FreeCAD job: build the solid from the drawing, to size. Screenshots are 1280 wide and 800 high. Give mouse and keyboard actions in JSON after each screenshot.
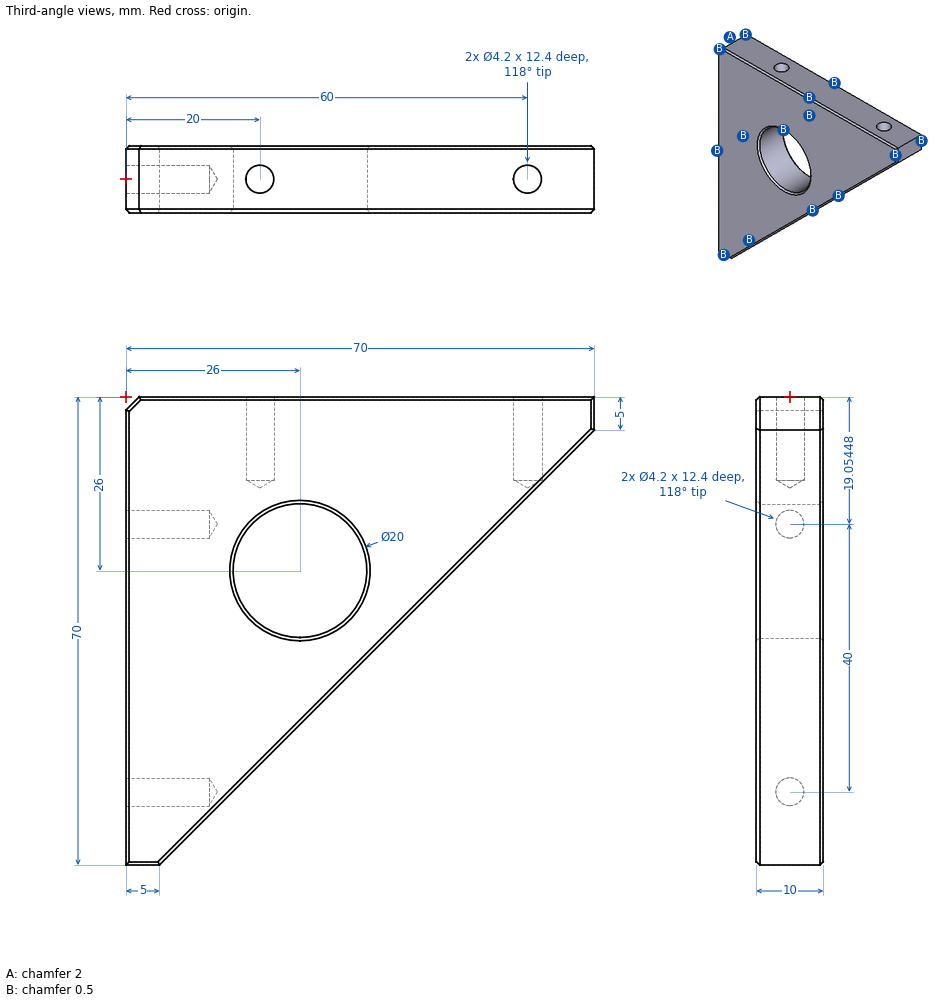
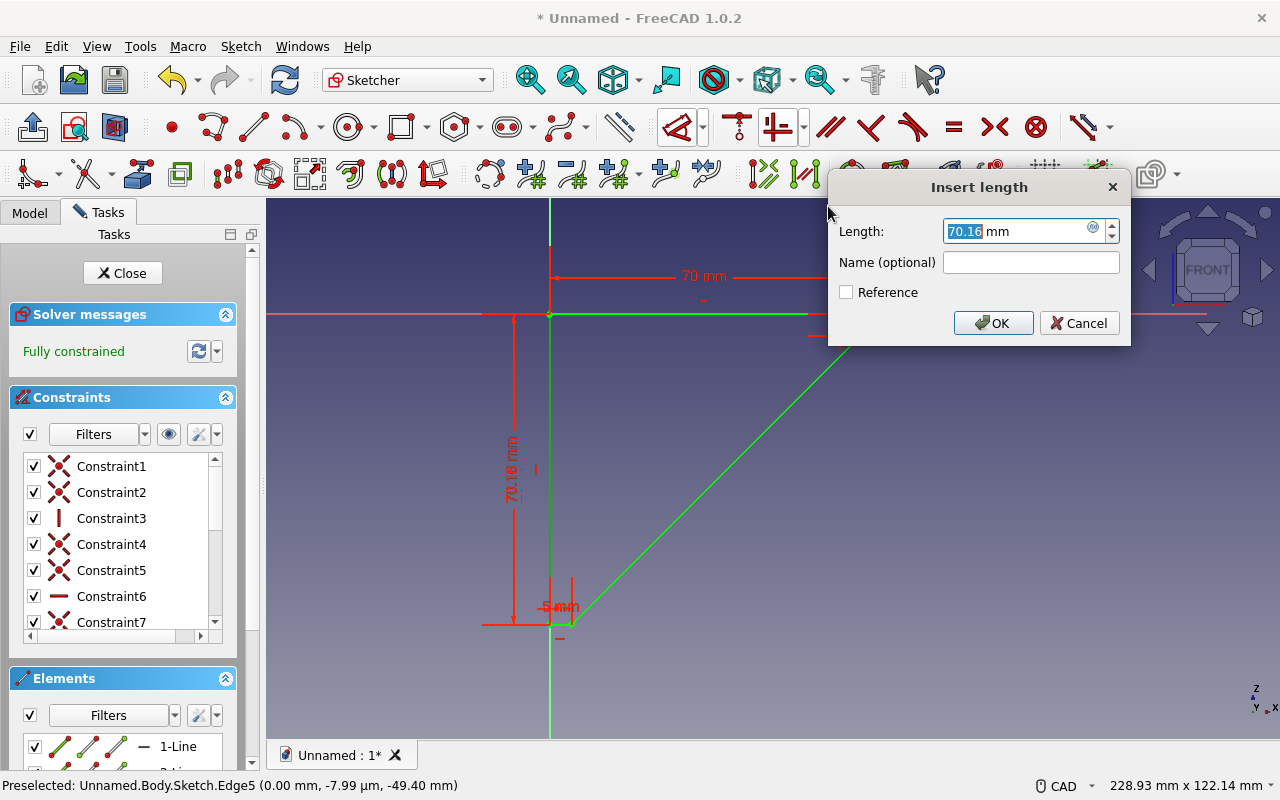
{"action": "type", "text": "70"}
{"action": "key", "text": "Return"}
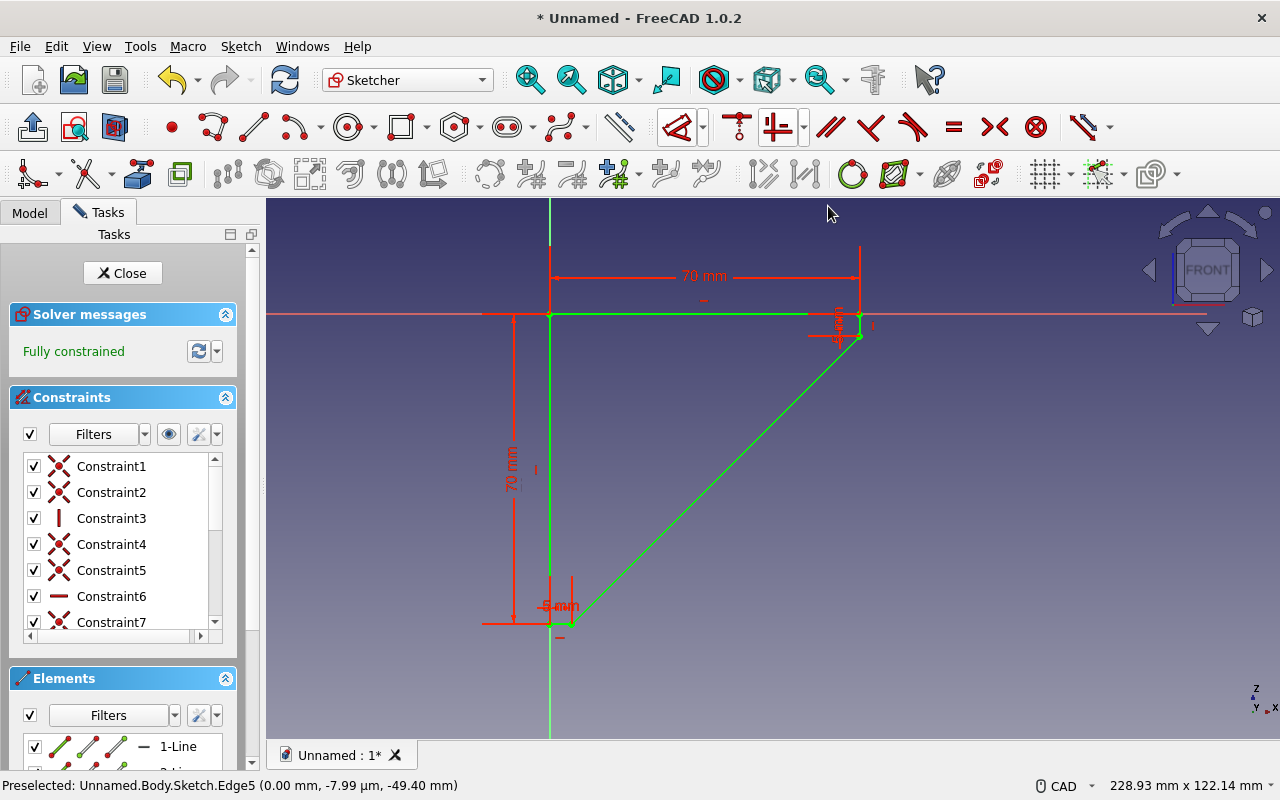
{"action": "left_click", "coordinate": [123, 273]}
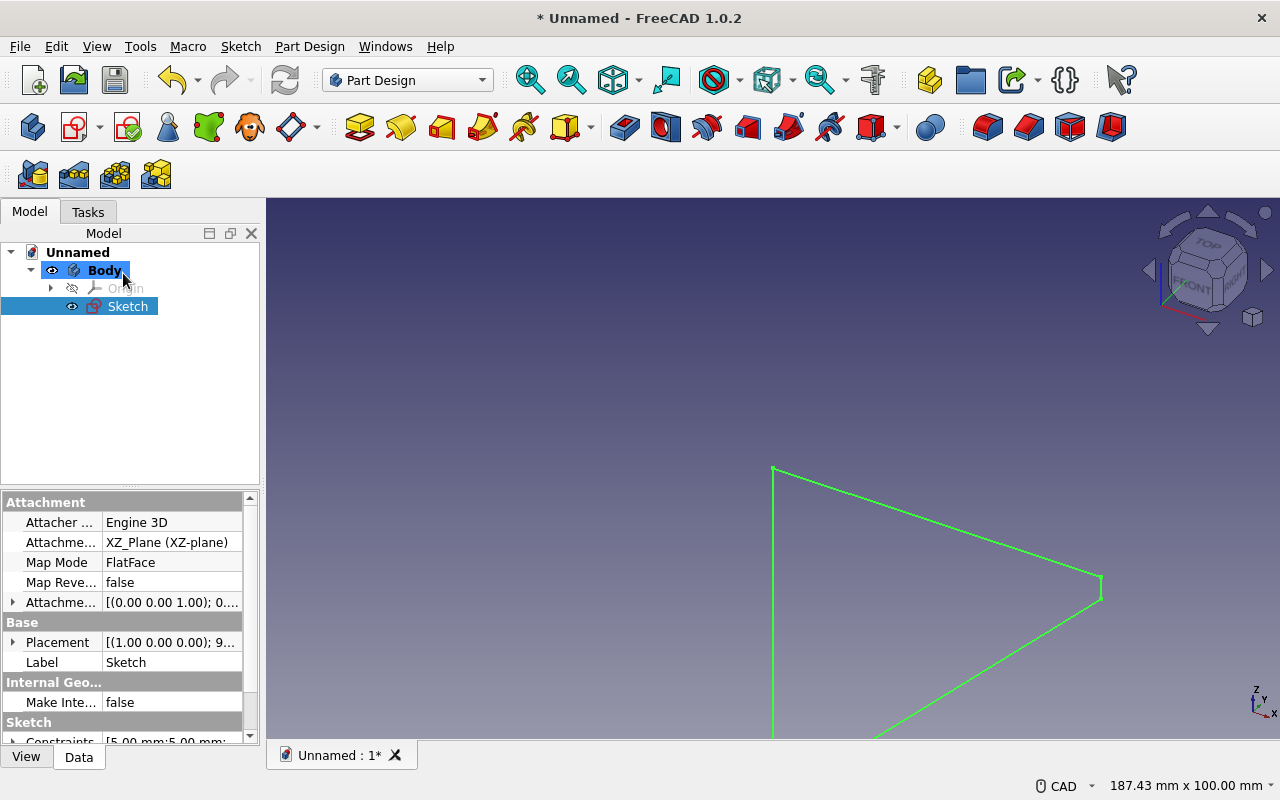
{"action": "left_click", "coordinate": [360, 128]}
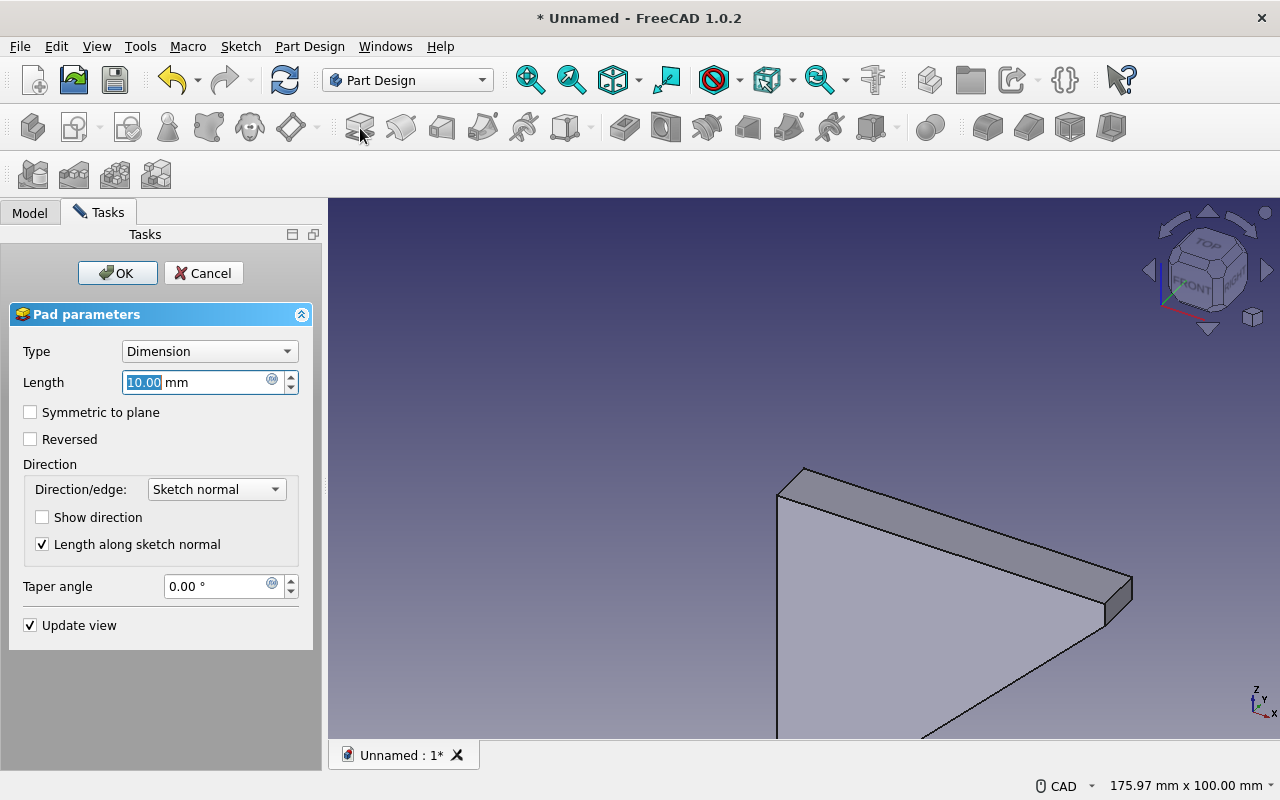
{"action": "type", "text": "10"}
{"action": "key", "text": "Tab"}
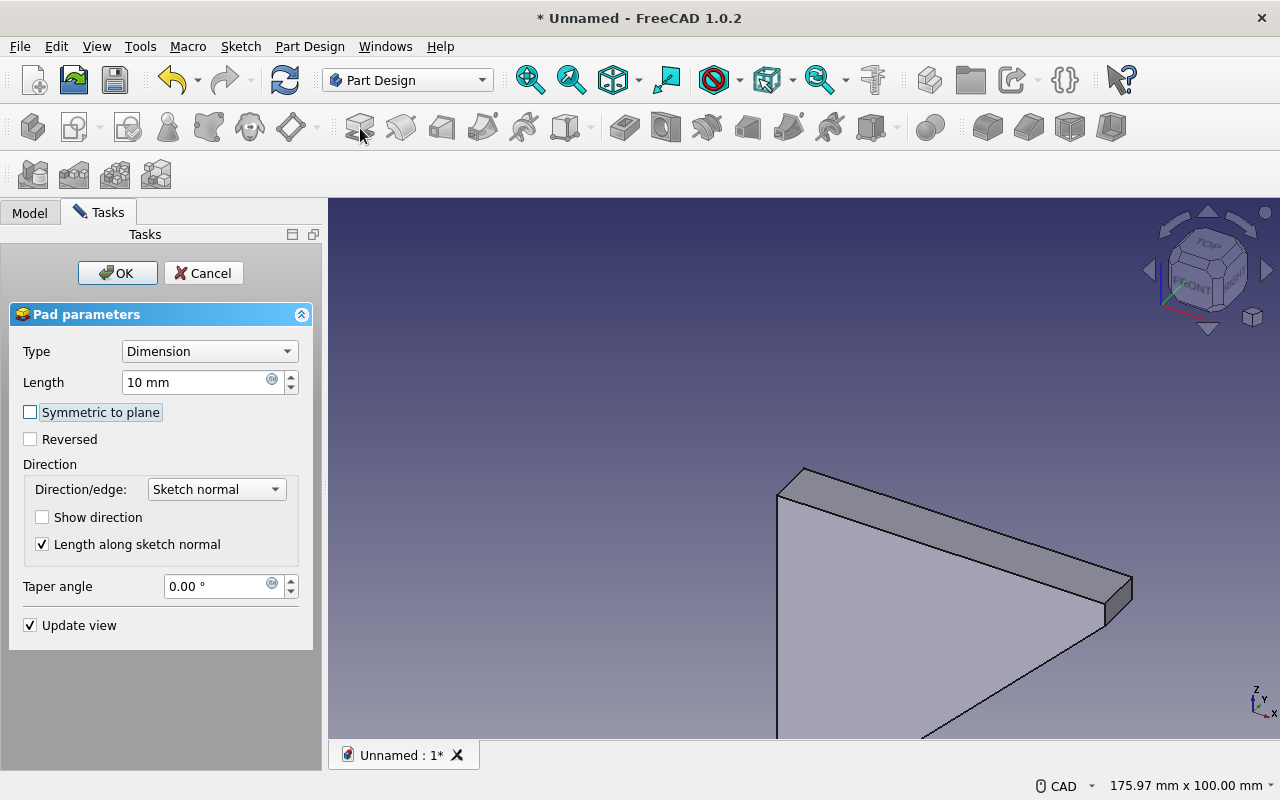
{"action": "left_click", "coordinate": [31, 412]}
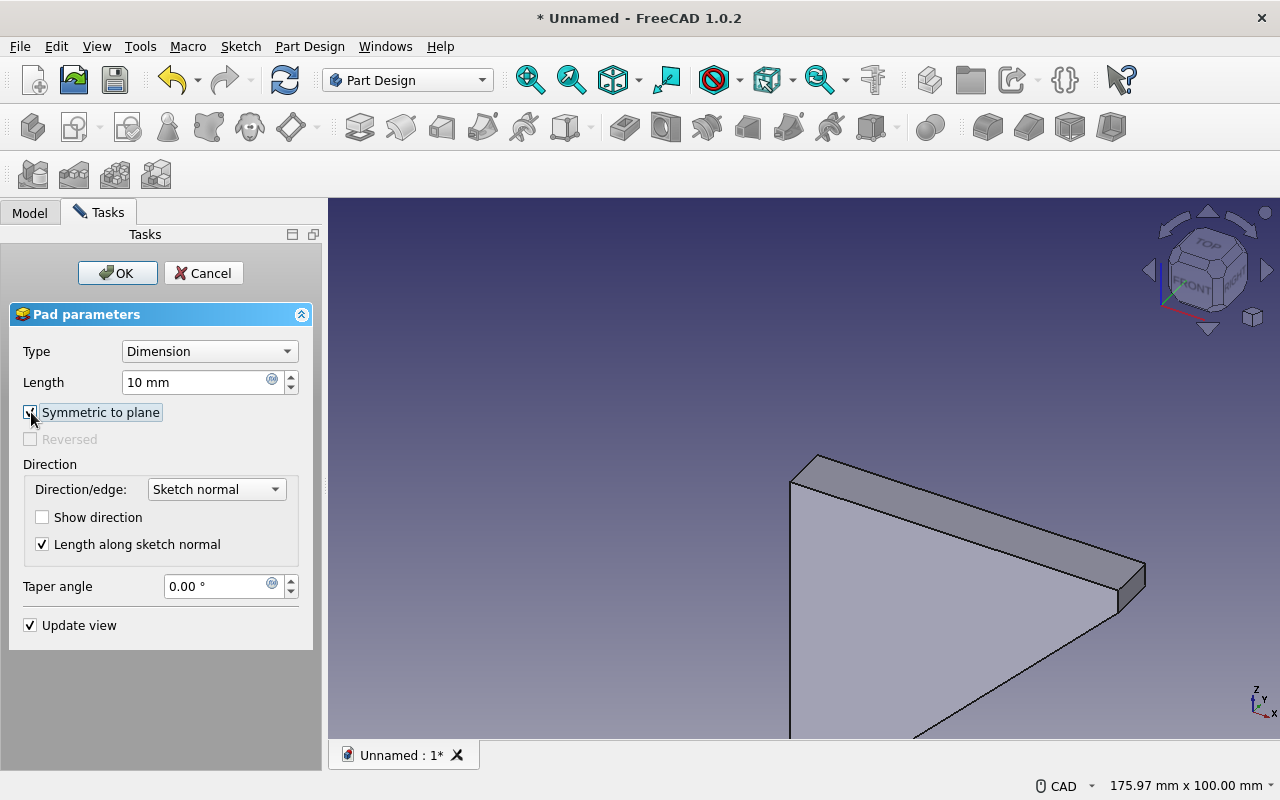
{"action": "left_click", "coordinate": [118, 273]}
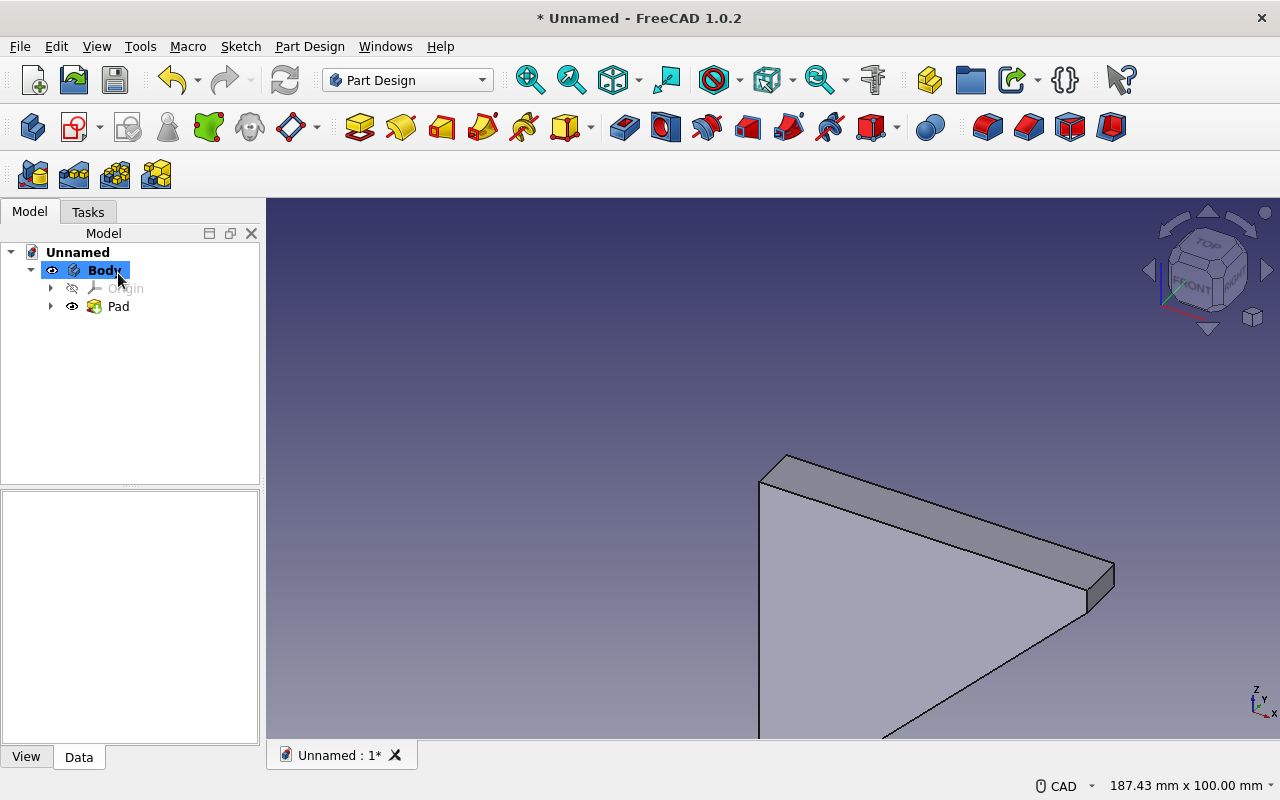
{"action": "left_click", "coordinate": [531, 80]}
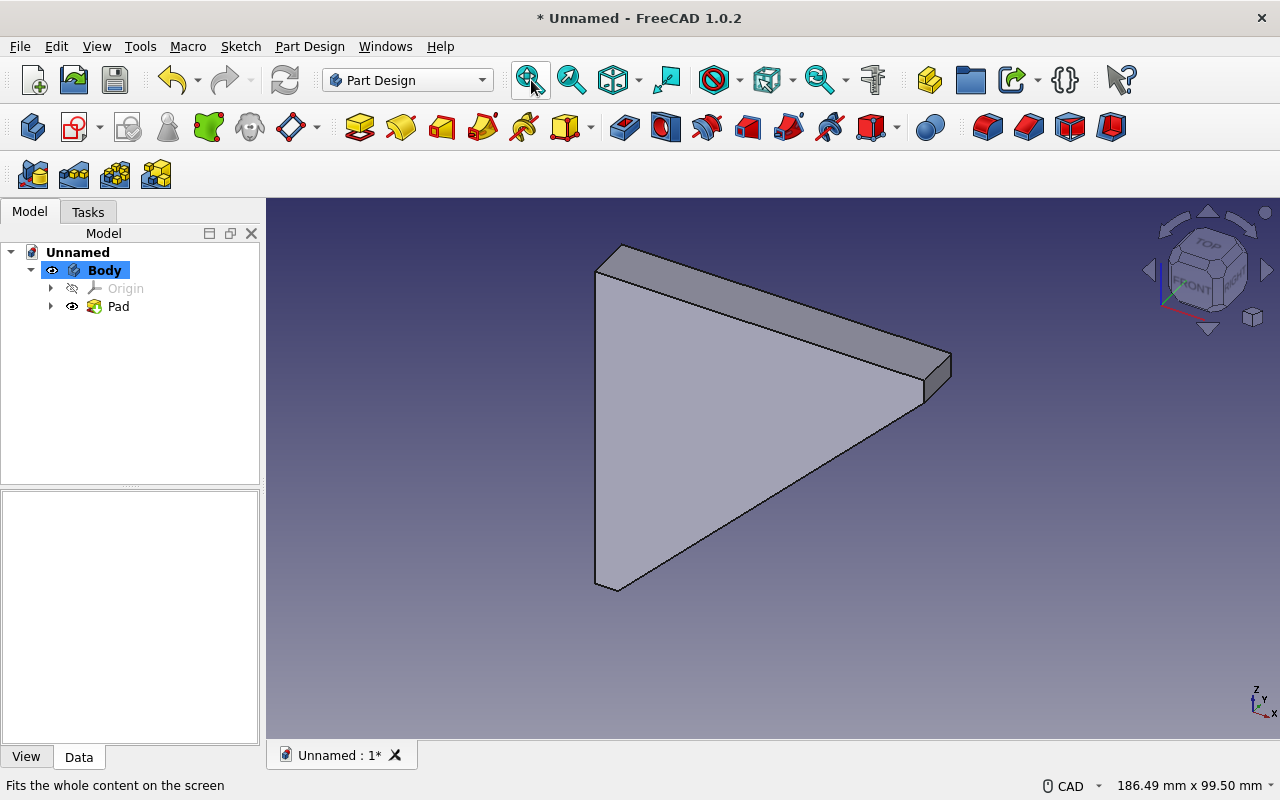
{"action": "key", "text": "0"}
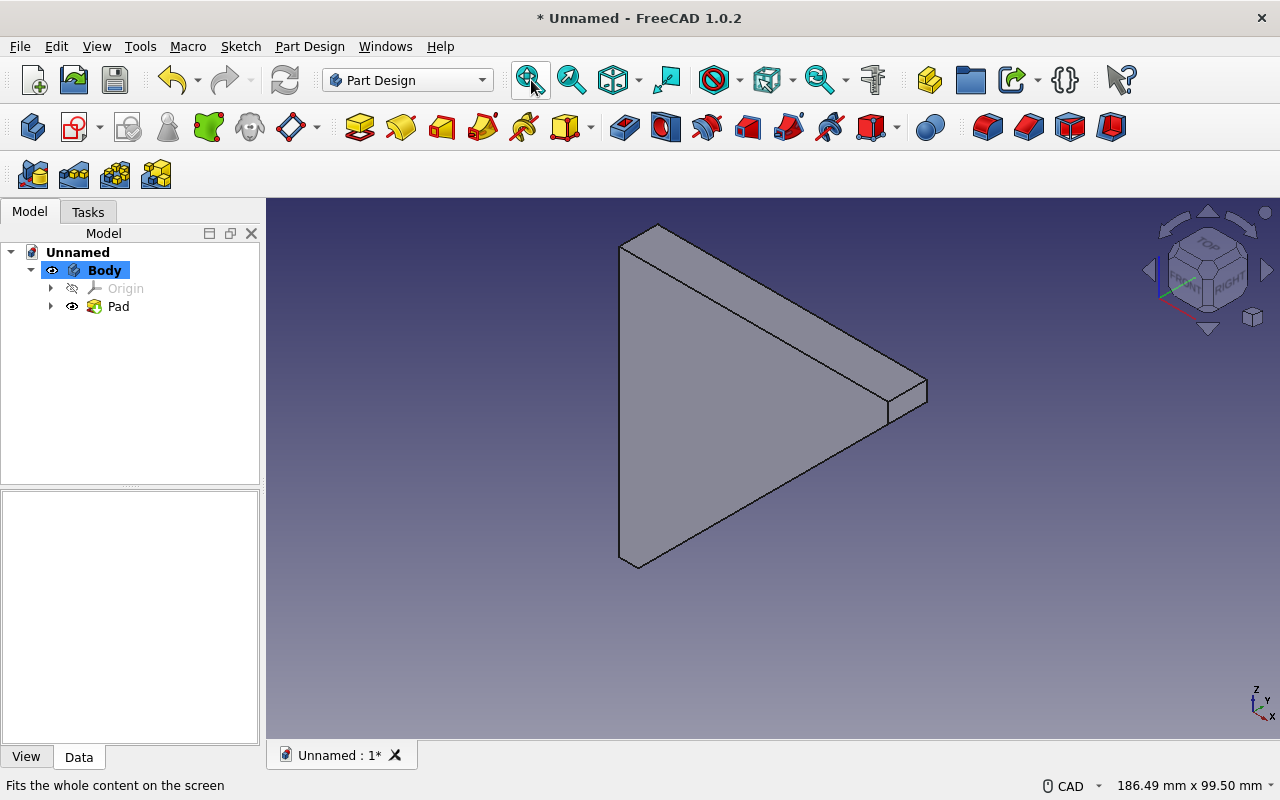
{"action": "key", "text": "2"}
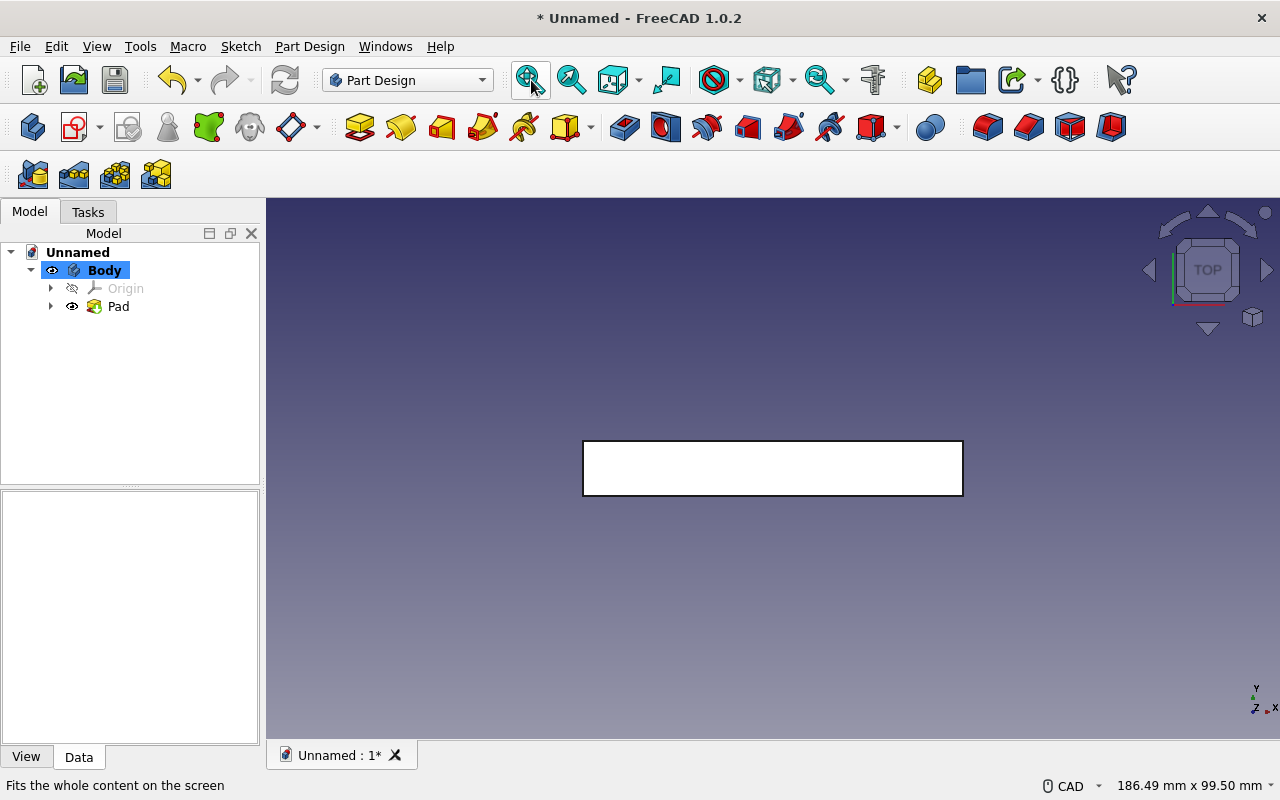
{"action": "left_click", "coordinate": [531, 80]}